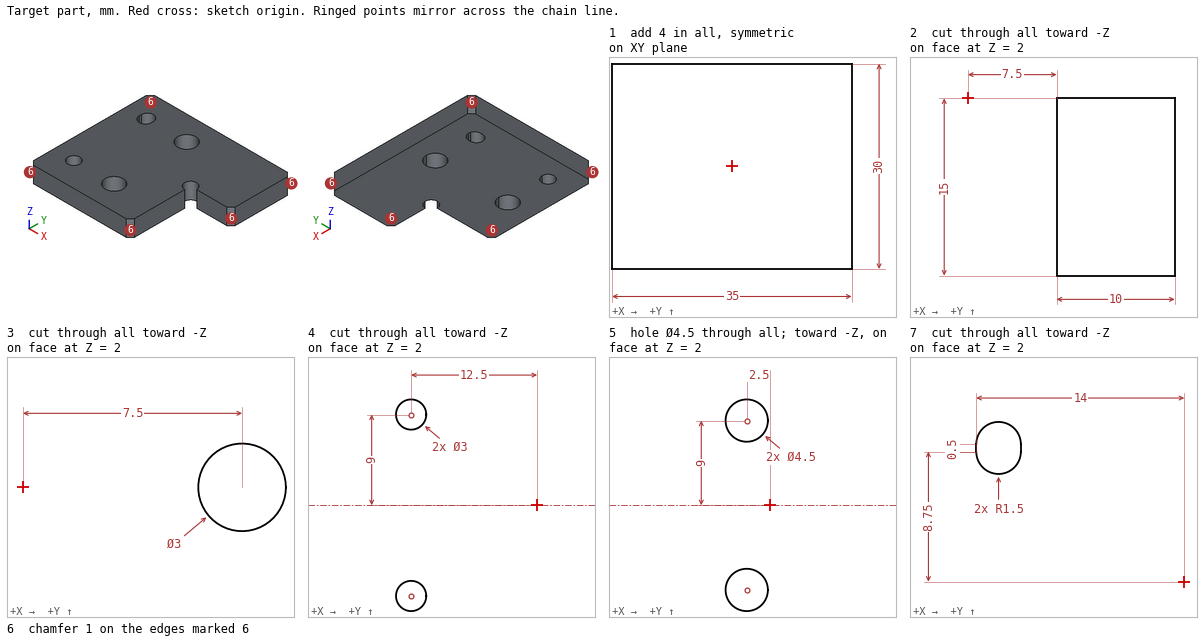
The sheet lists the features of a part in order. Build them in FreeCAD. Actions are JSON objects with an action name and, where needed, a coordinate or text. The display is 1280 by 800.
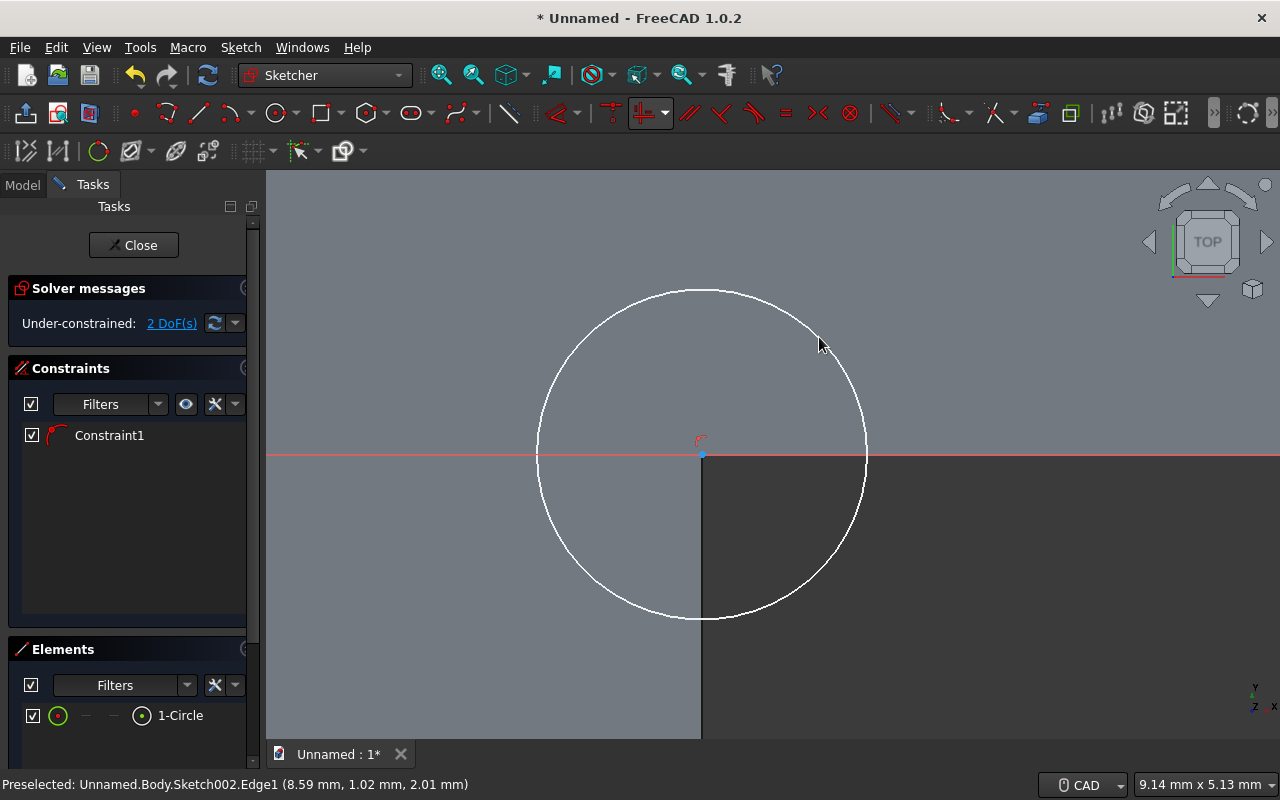
{"action": "key", "text": "d"}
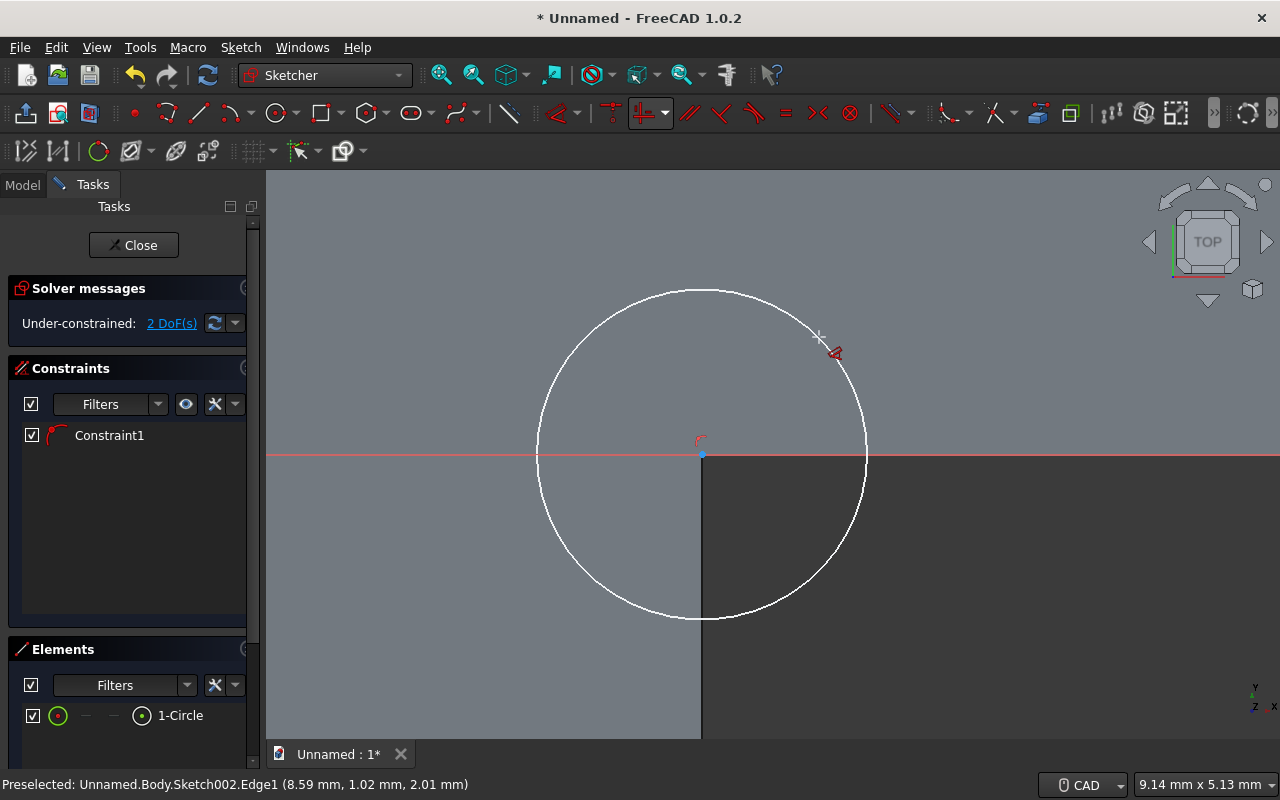
{"action": "left_click", "coordinate": [818, 337]}
{"action": "left_click", "coordinate": [840, 314]}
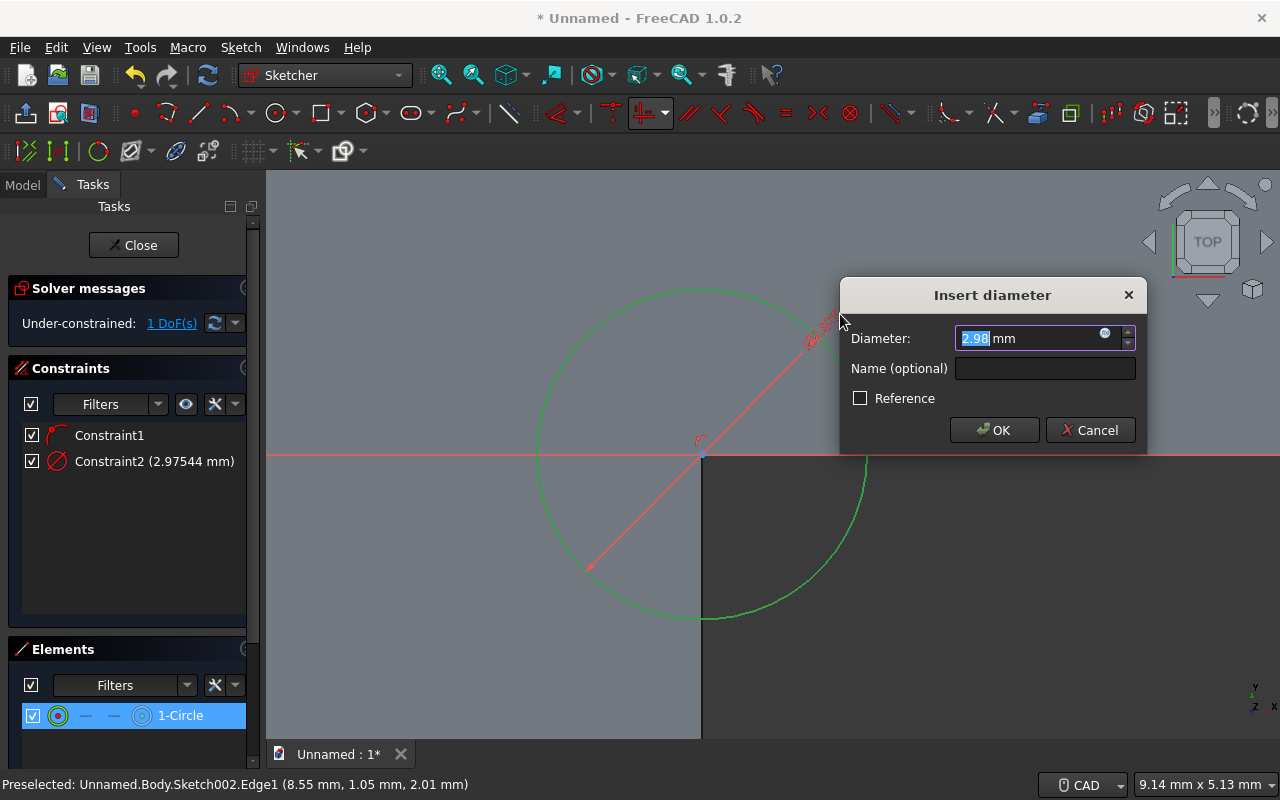
{"action": "type", "text": "3"}
{"action": "key", "text": "Return"}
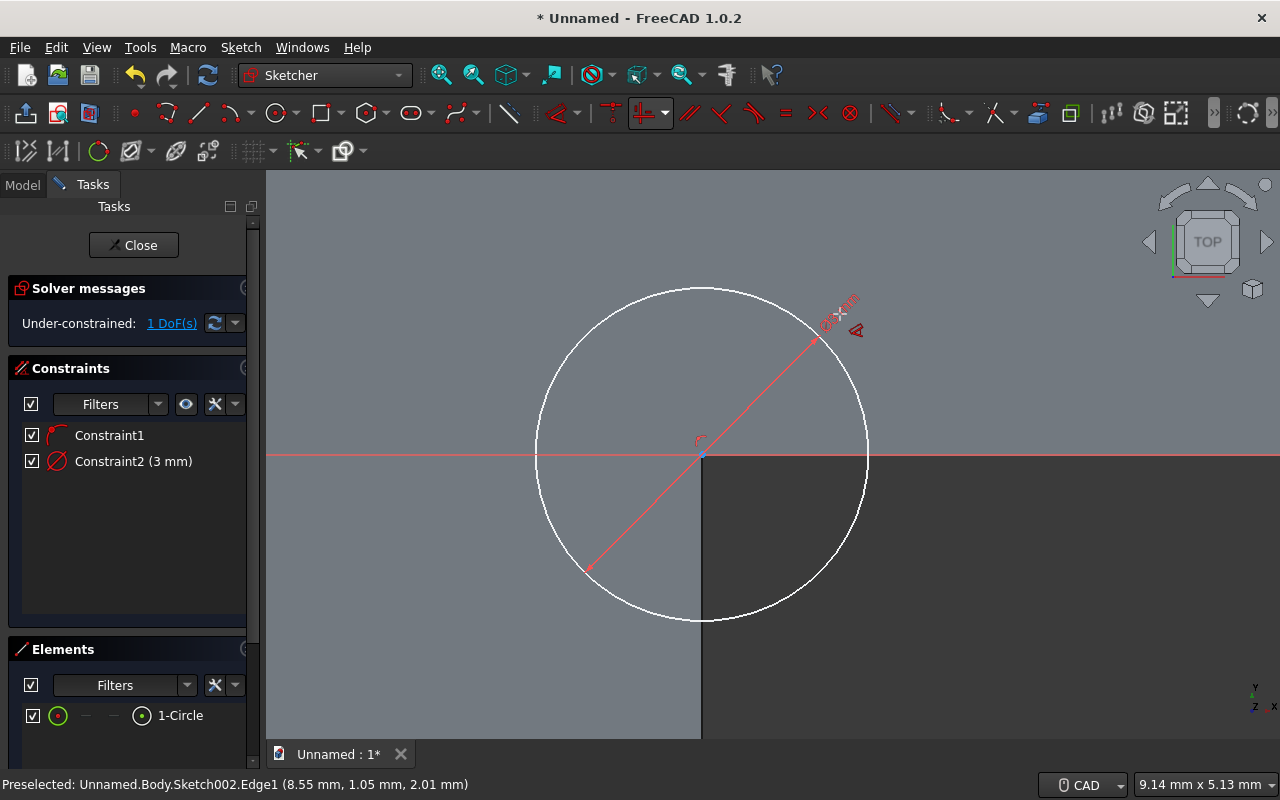
{"action": "left_click", "coordinate": [702, 454]}
{"action": "left_click", "coordinate": [498, 488]}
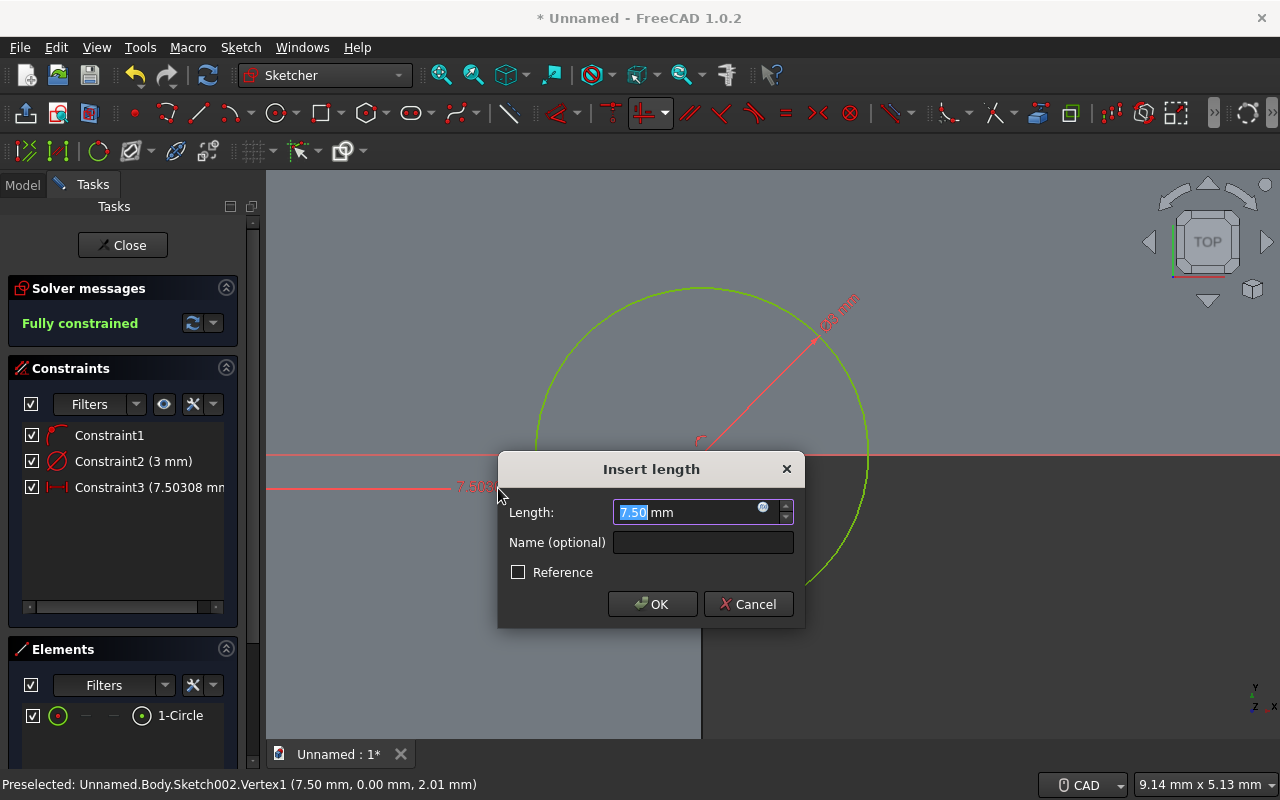
{"action": "type", "text": "7.5"}
{"action": "key", "text": "Return"}
{"action": "key", "text": "Escape"}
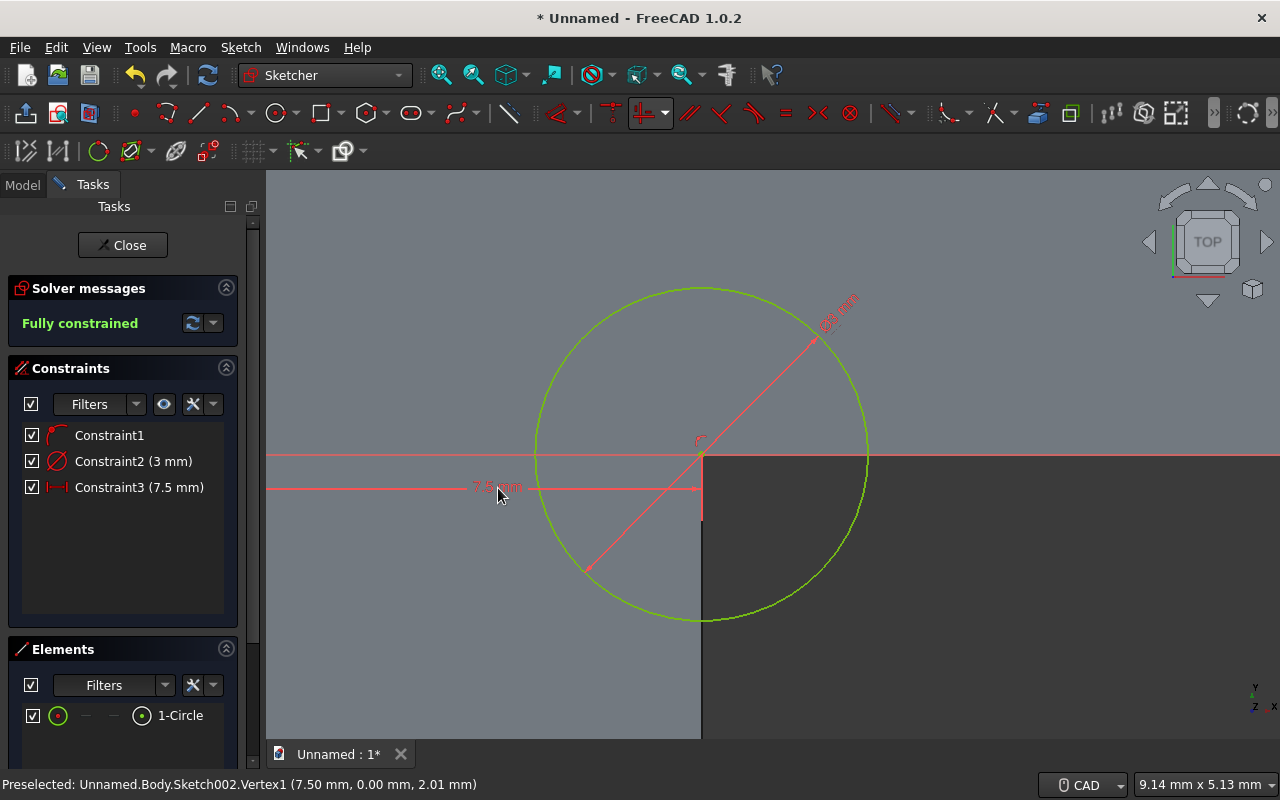
{"action": "left_click", "coordinate": [123, 245]}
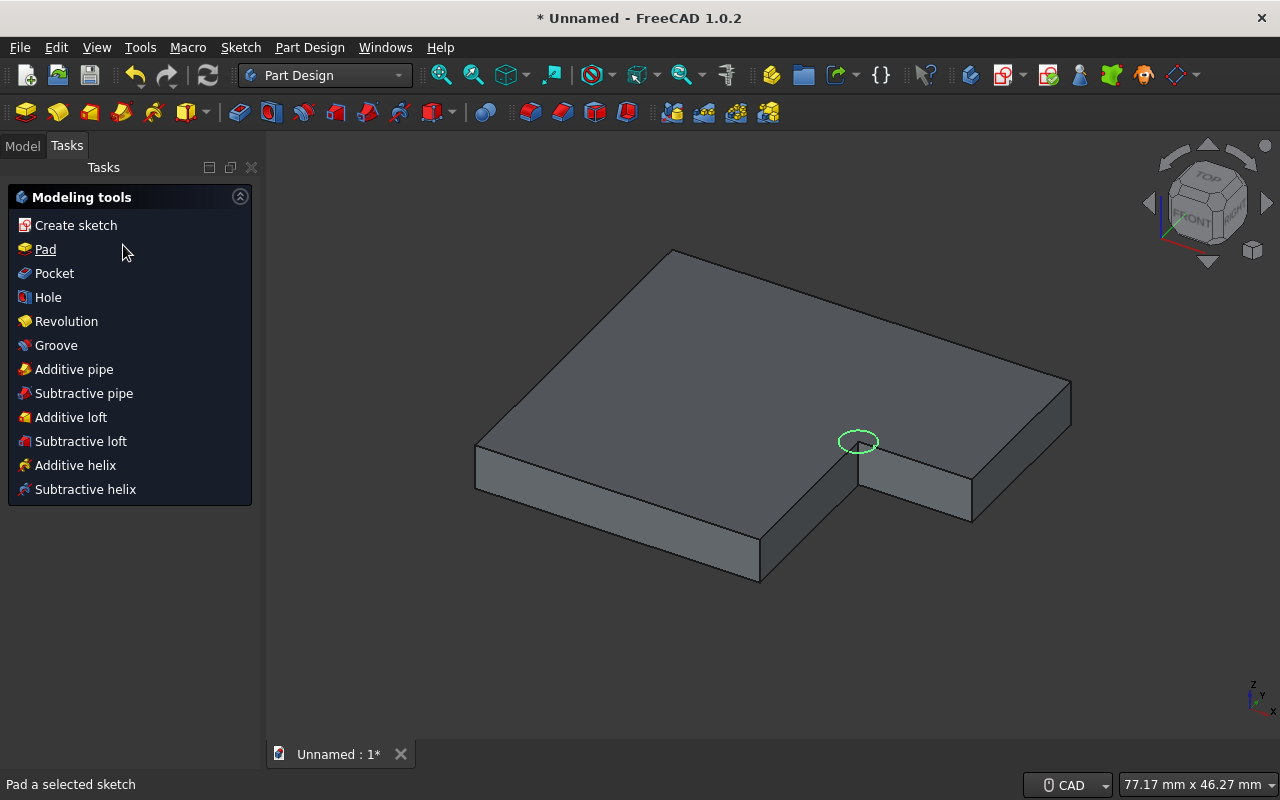
{"action": "left_click", "coordinate": [240, 112]}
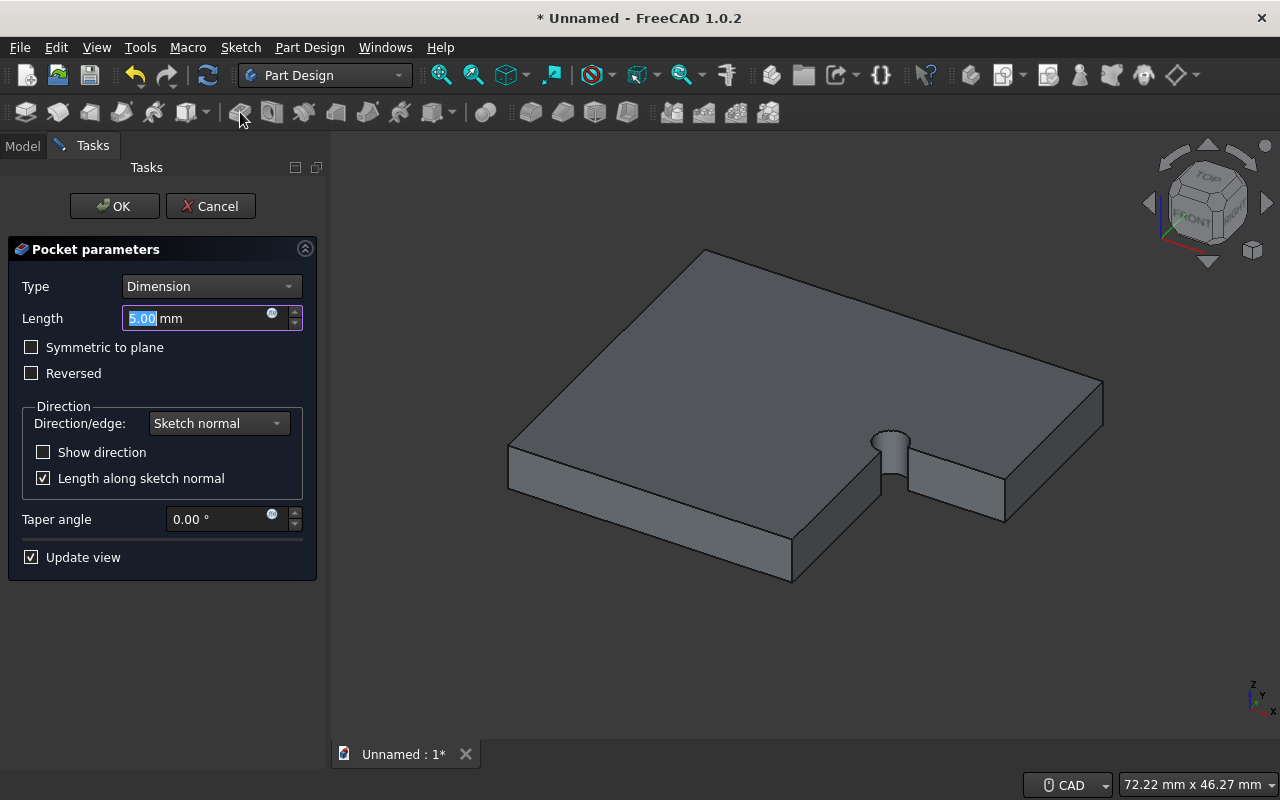
{"action": "left_click", "coordinate": [212, 286]}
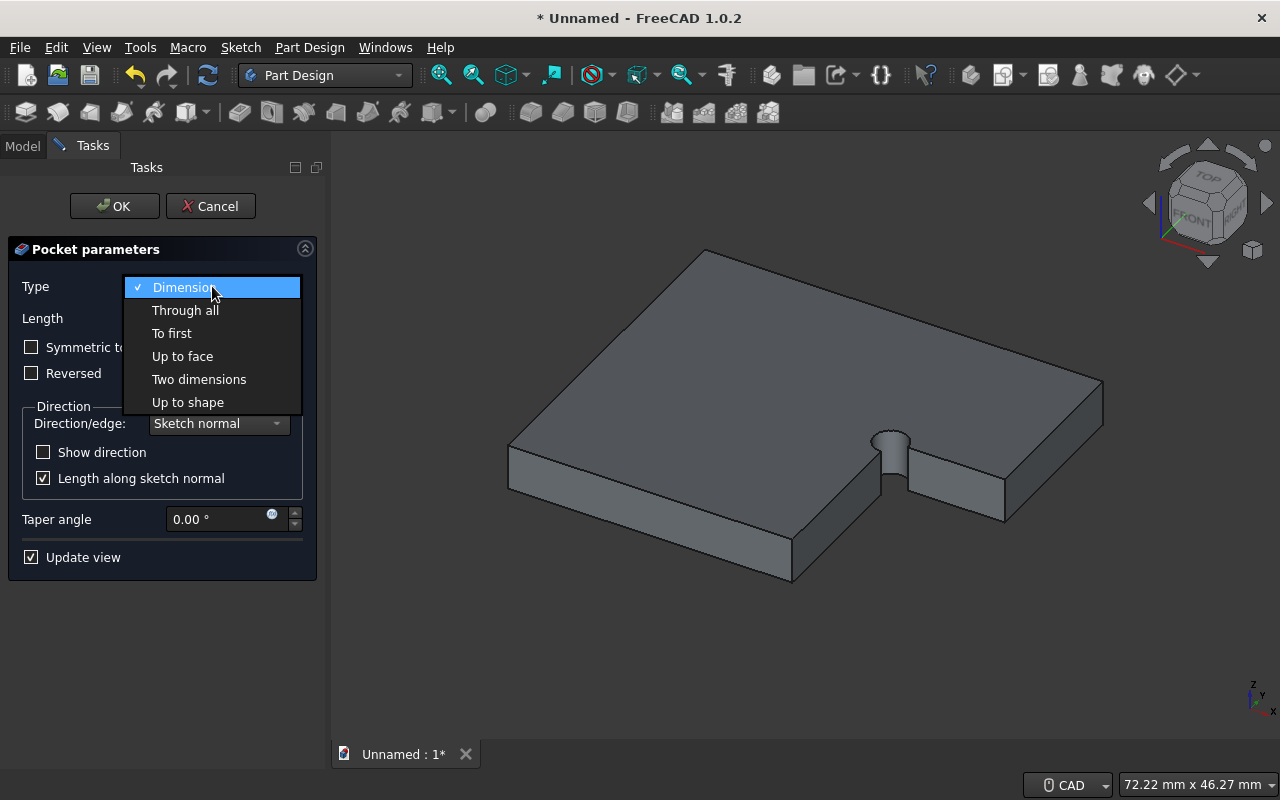
{"action": "left_click", "coordinate": [212, 310]}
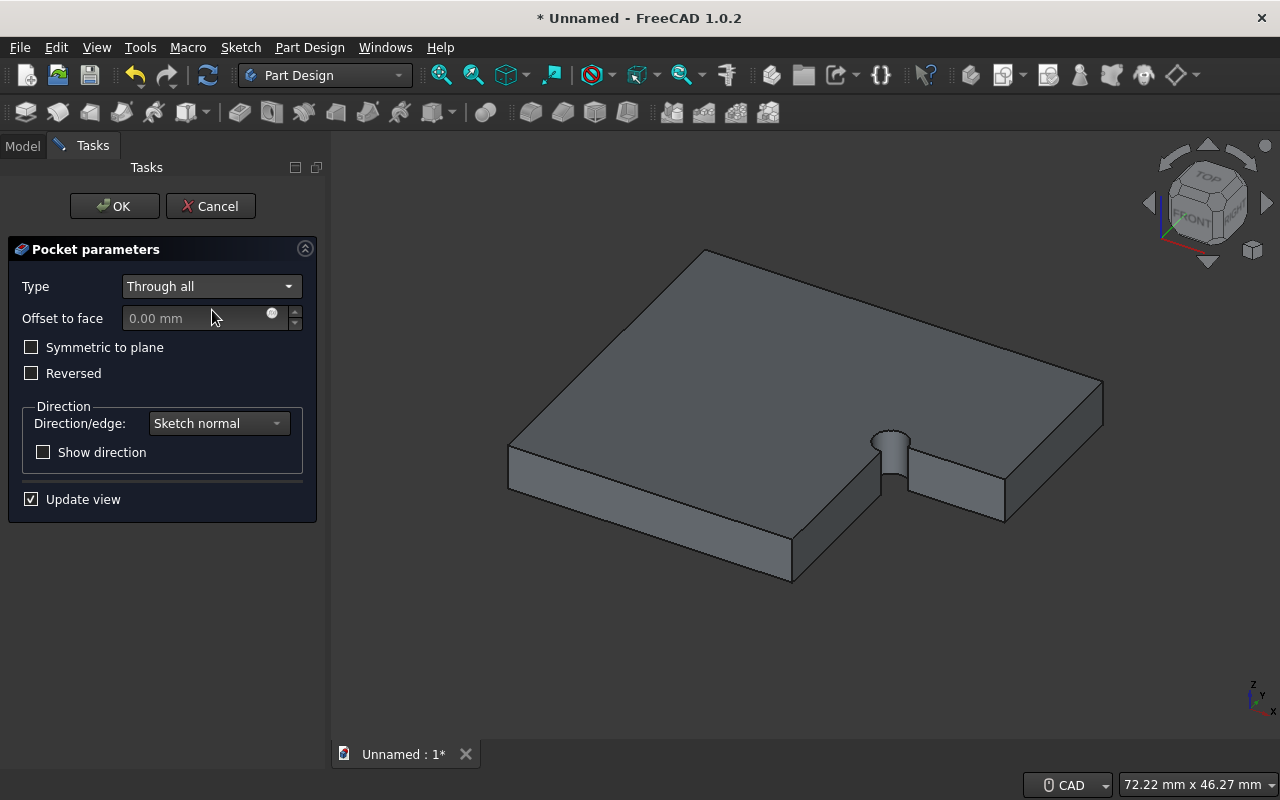
{"action": "left_click", "coordinate": [115, 206]}